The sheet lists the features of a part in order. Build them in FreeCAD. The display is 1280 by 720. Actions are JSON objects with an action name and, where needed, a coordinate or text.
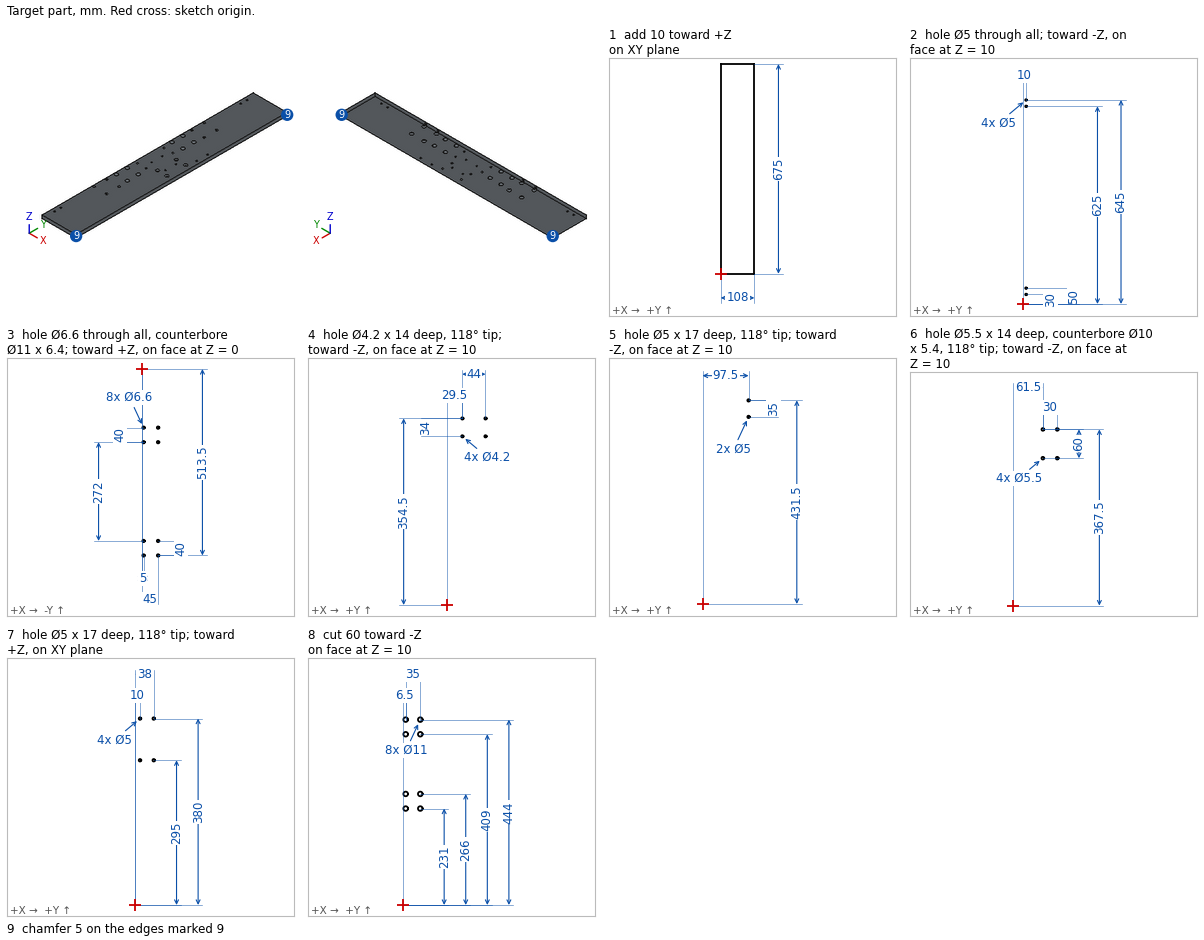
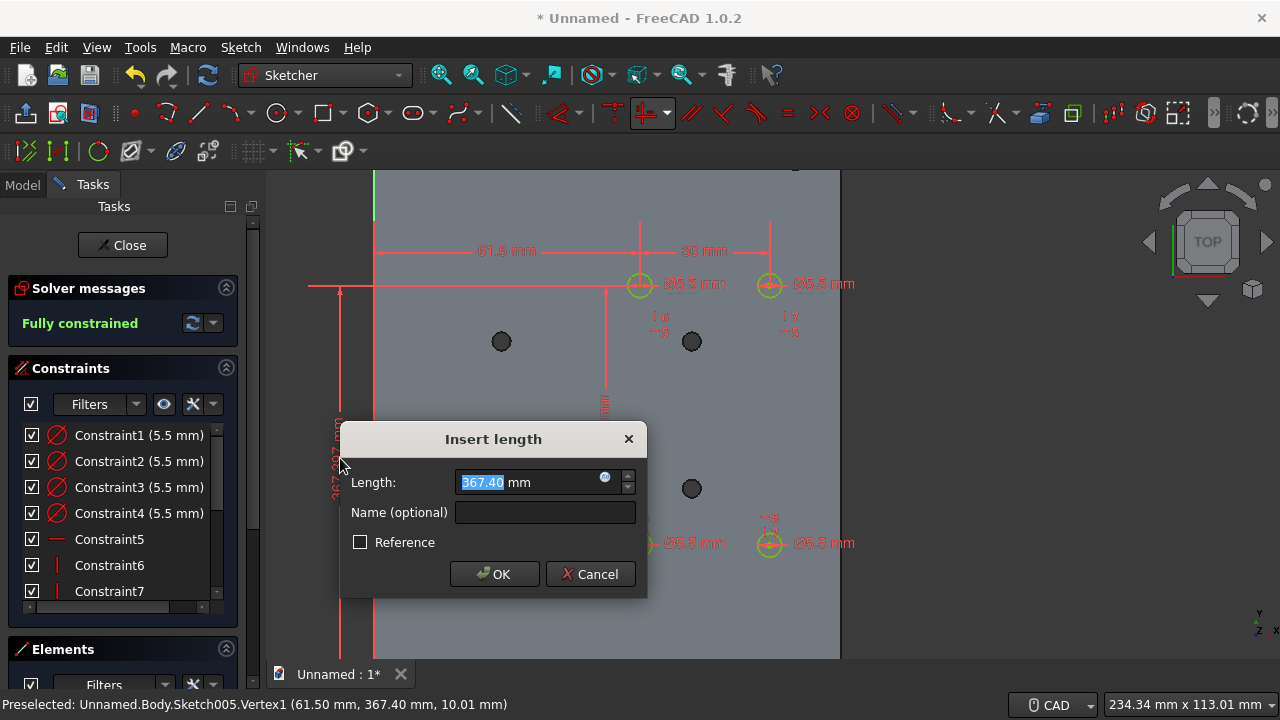
{"action": "type", "text": "367.5"}
{"action": "key", "text": "Return"}
{"action": "key", "text": "Escape"}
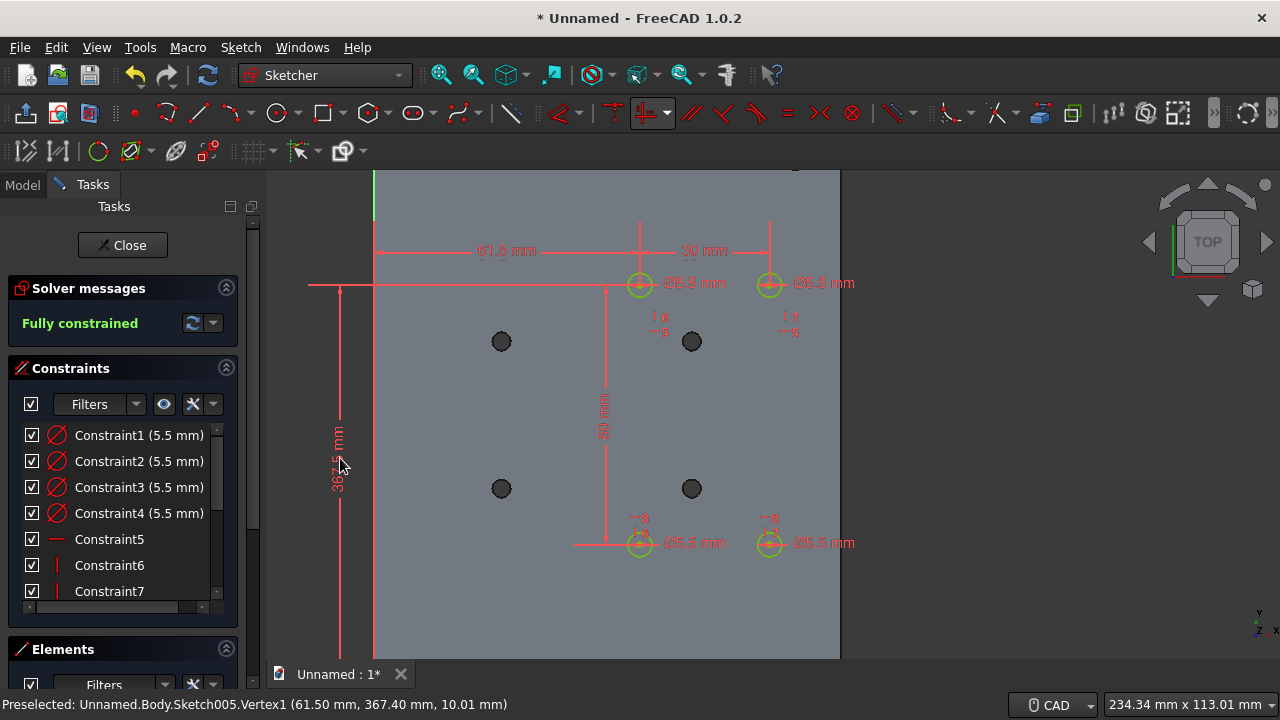
{"action": "left_click", "coordinate": [123, 245]}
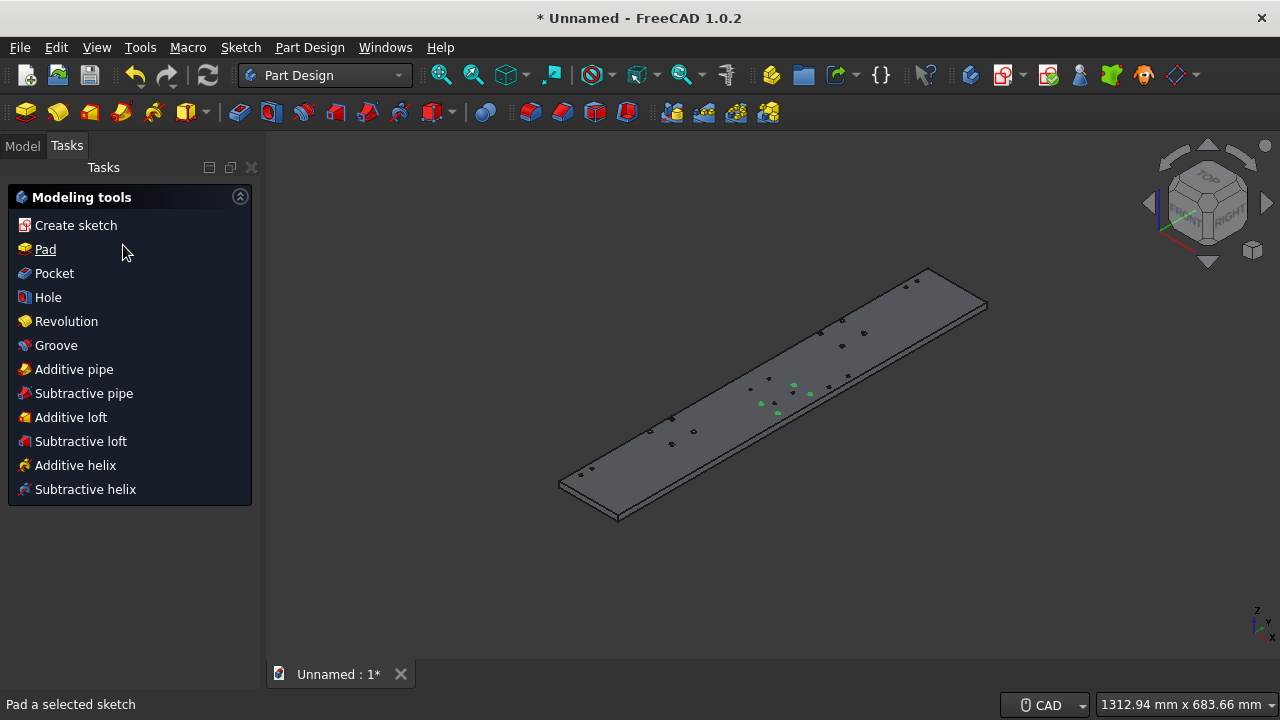
{"action": "left_click", "coordinate": [272, 112]}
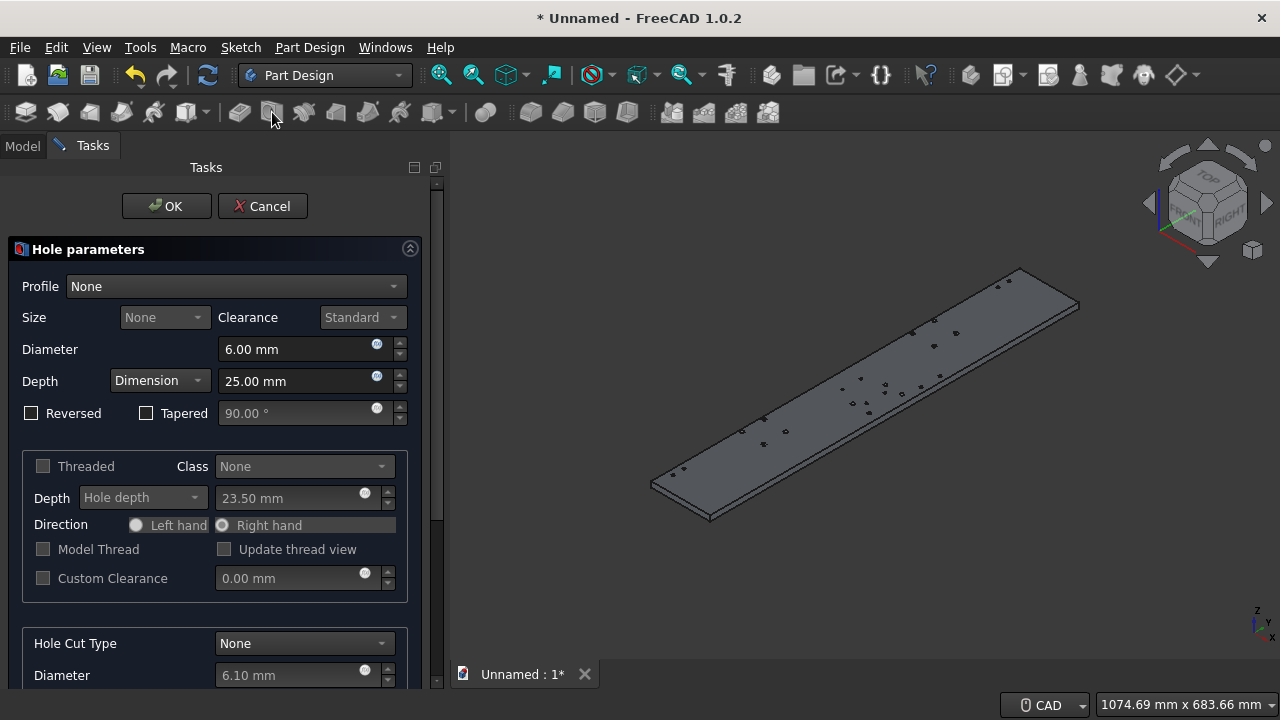
{"action": "triple_click", "coordinate": [305, 349]}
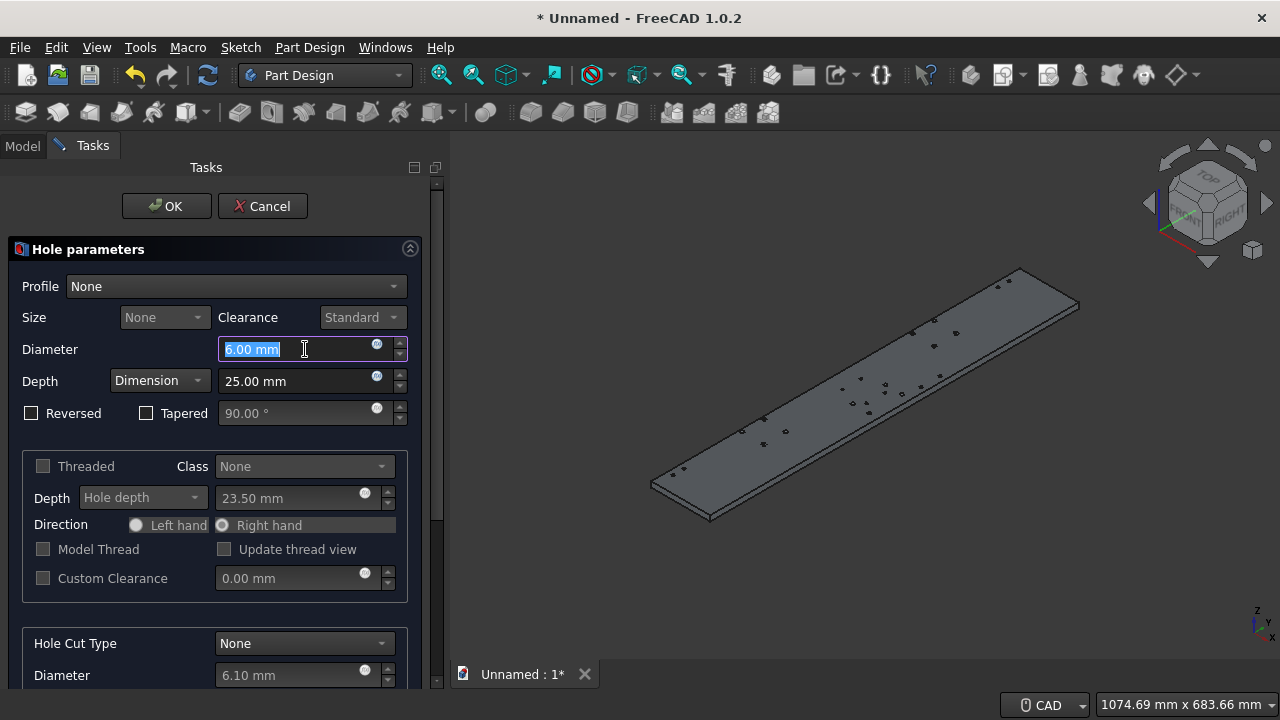
{"action": "type", "text": "5.5"}
{"action": "key", "text": "Tab"}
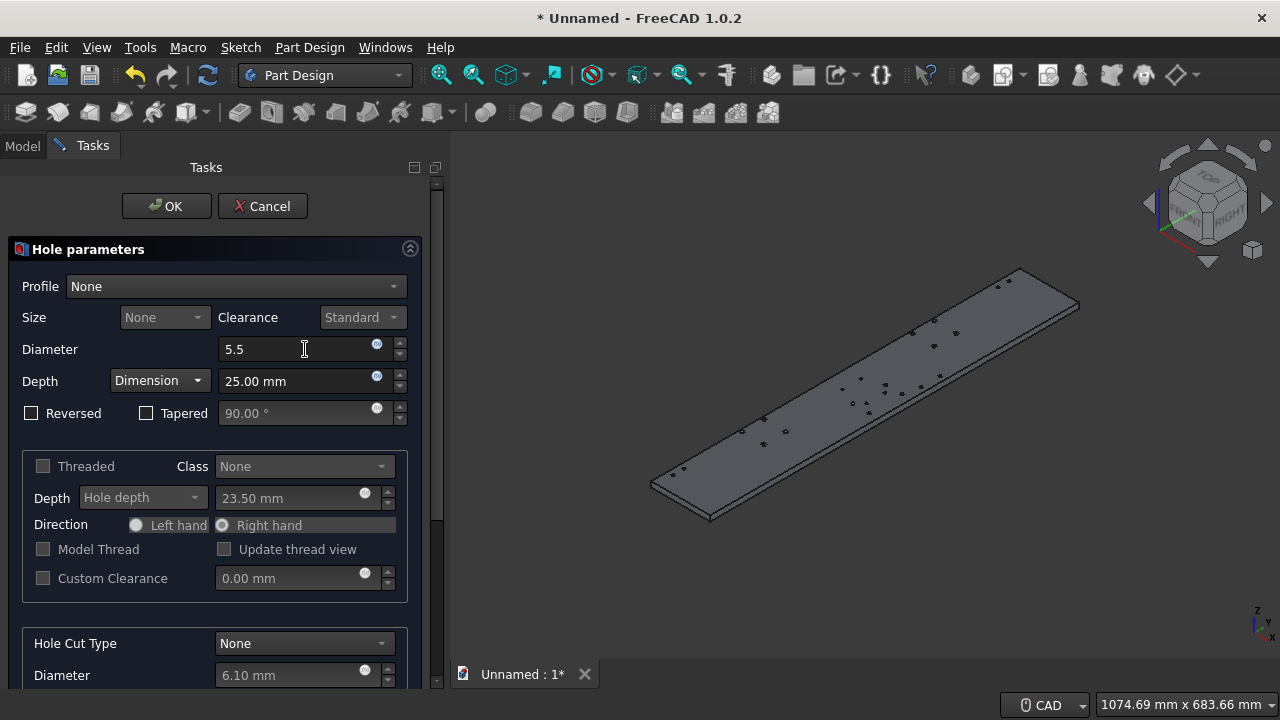
{"action": "triple_click", "coordinate": [305, 381]}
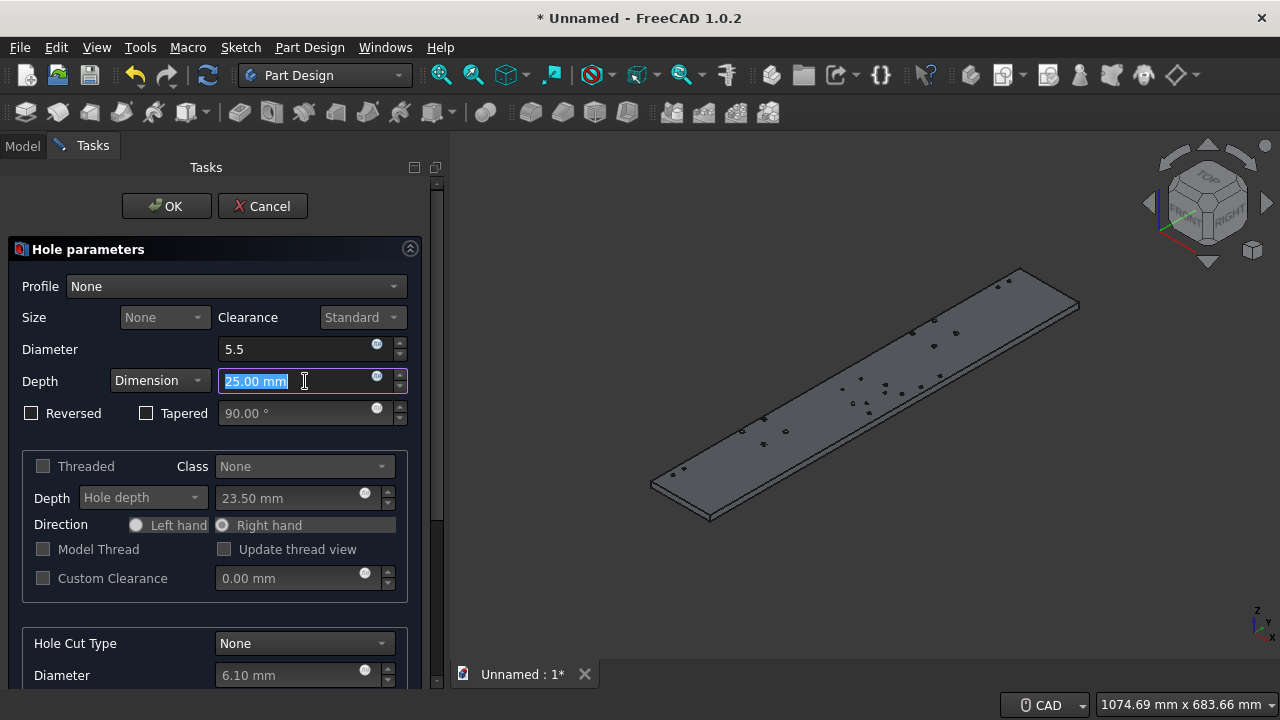
{"action": "type", "text": "14"}
{"action": "key", "text": "Tab"}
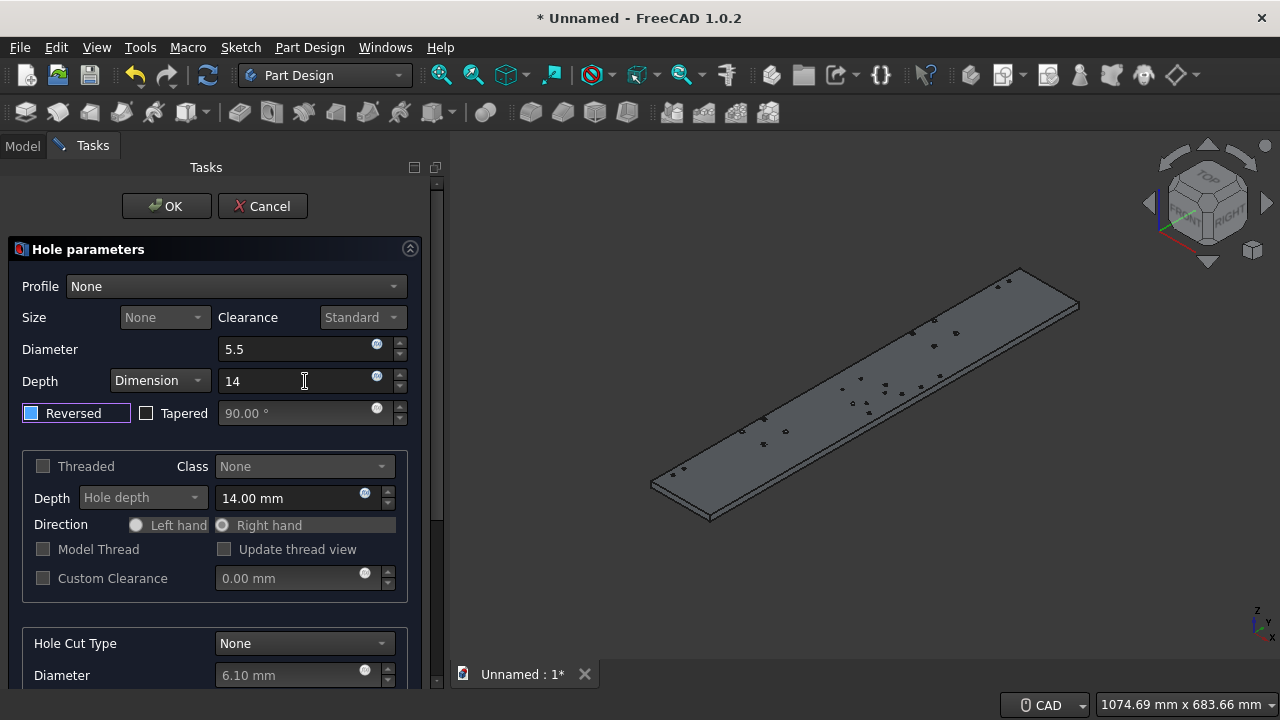
{"action": "left_click", "coordinate": [306, 644]}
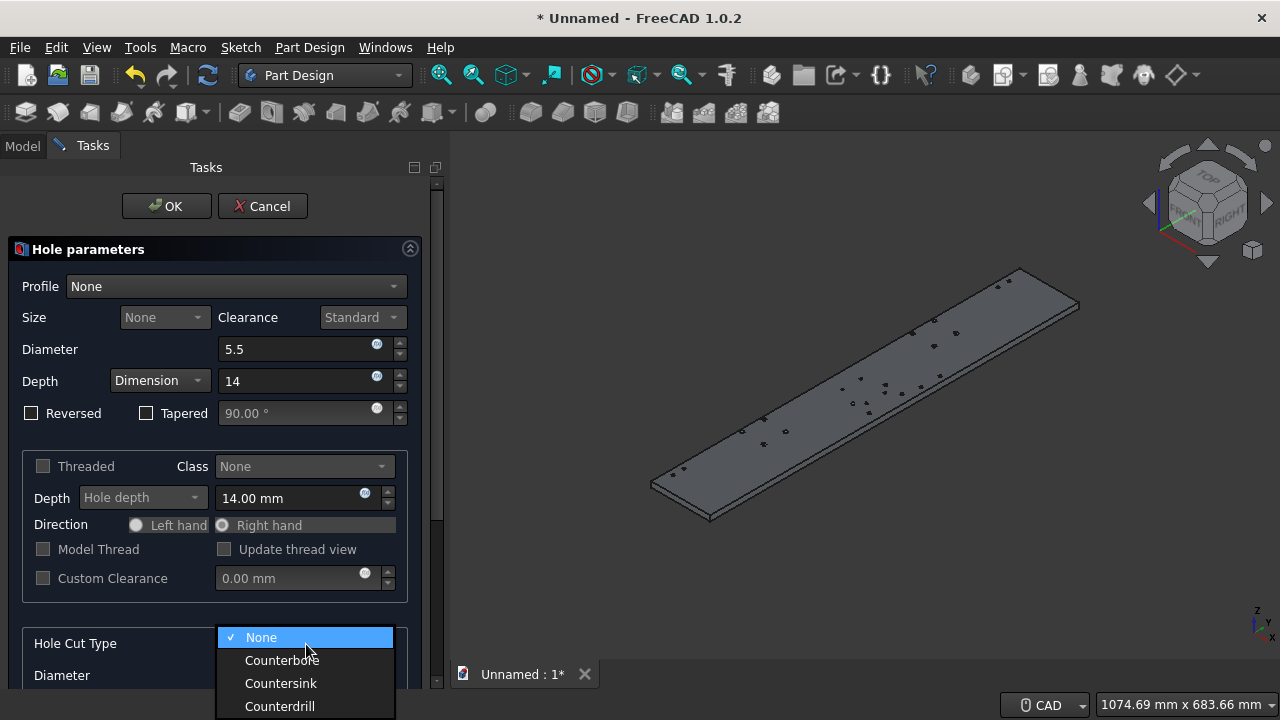
{"action": "left_click", "coordinate": [304, 660]}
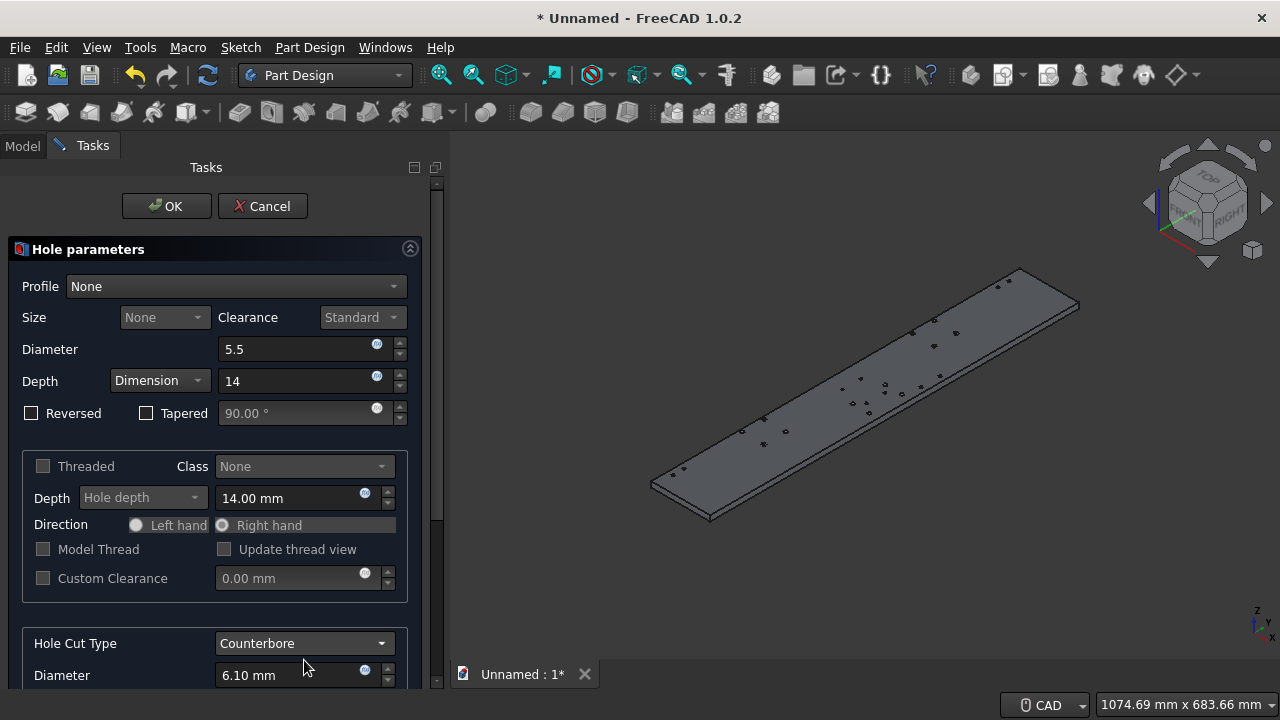
{"action": "triple_click", "coordinate": [298, 675]}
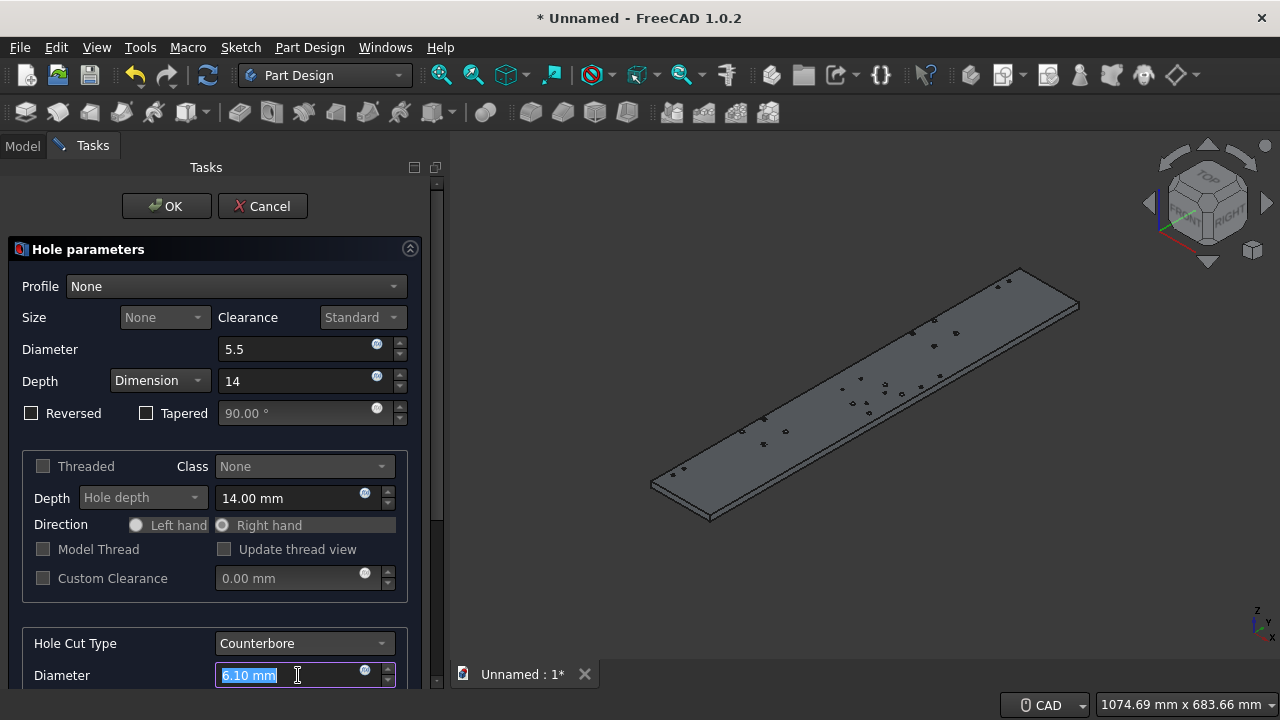
{"action": "type", "text": "10"}
{"action": "key", "text": "Tab"}